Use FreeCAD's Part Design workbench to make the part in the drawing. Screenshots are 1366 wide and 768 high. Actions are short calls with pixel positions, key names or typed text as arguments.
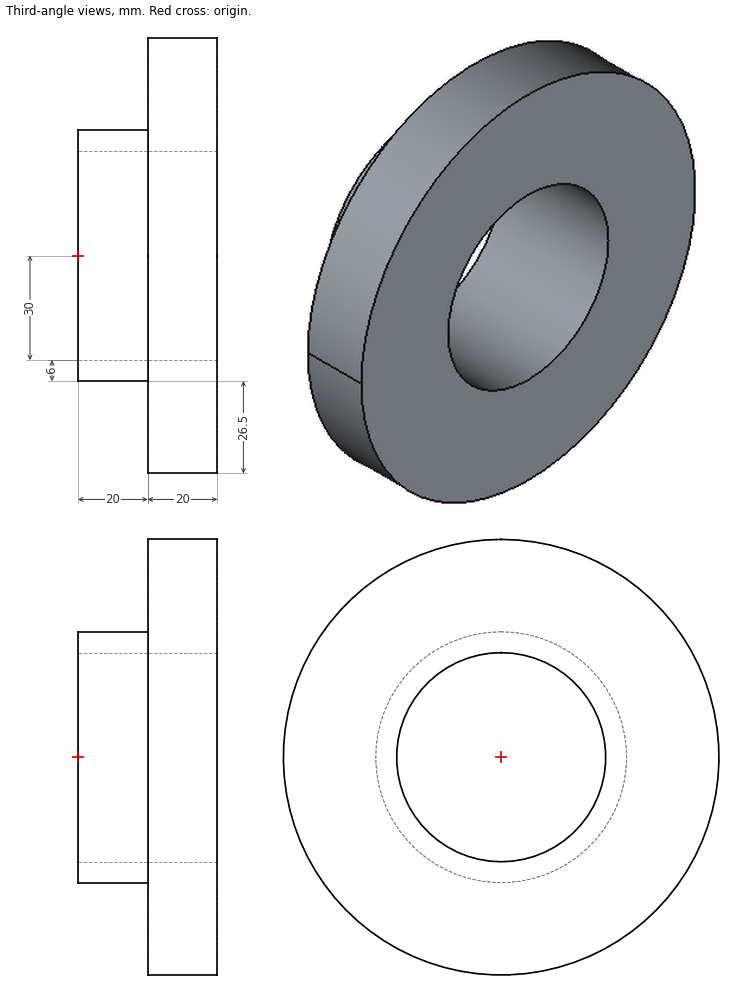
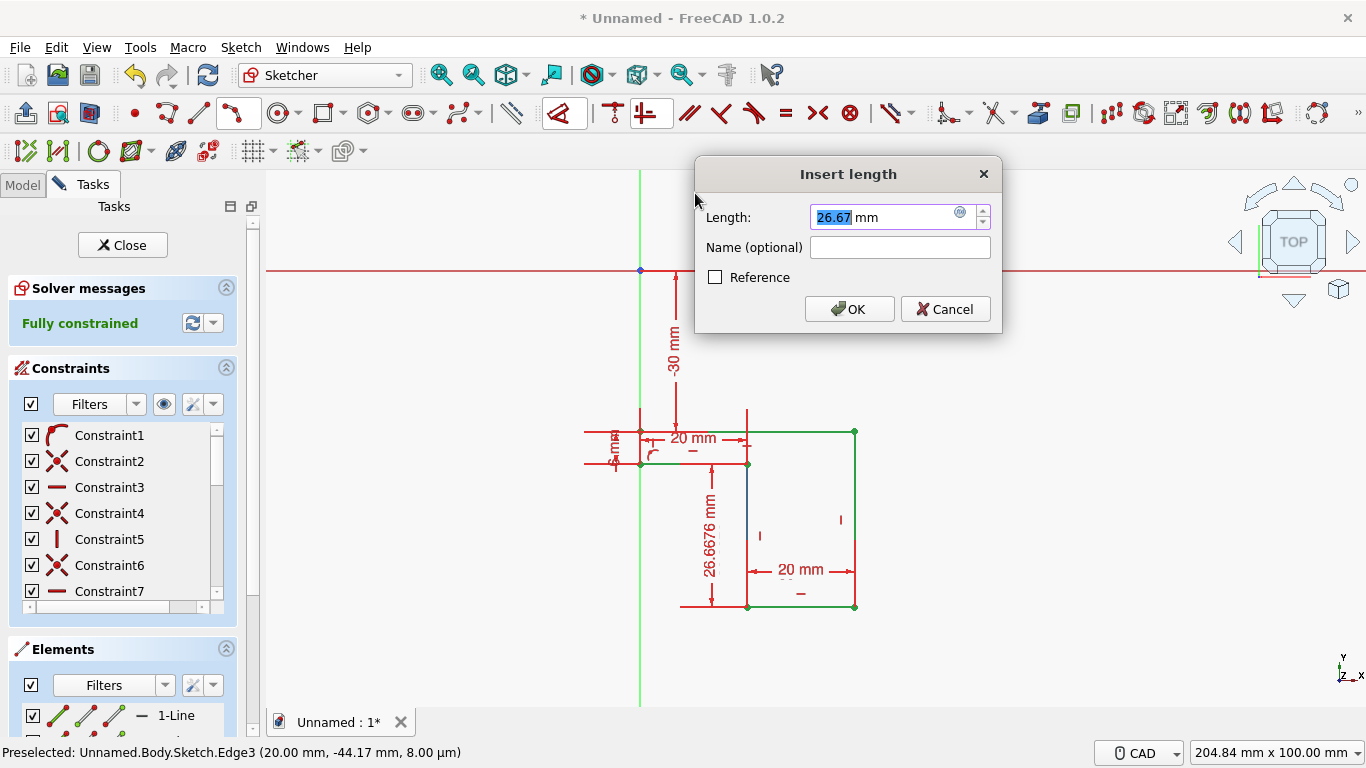
text(26.5)
key(Return)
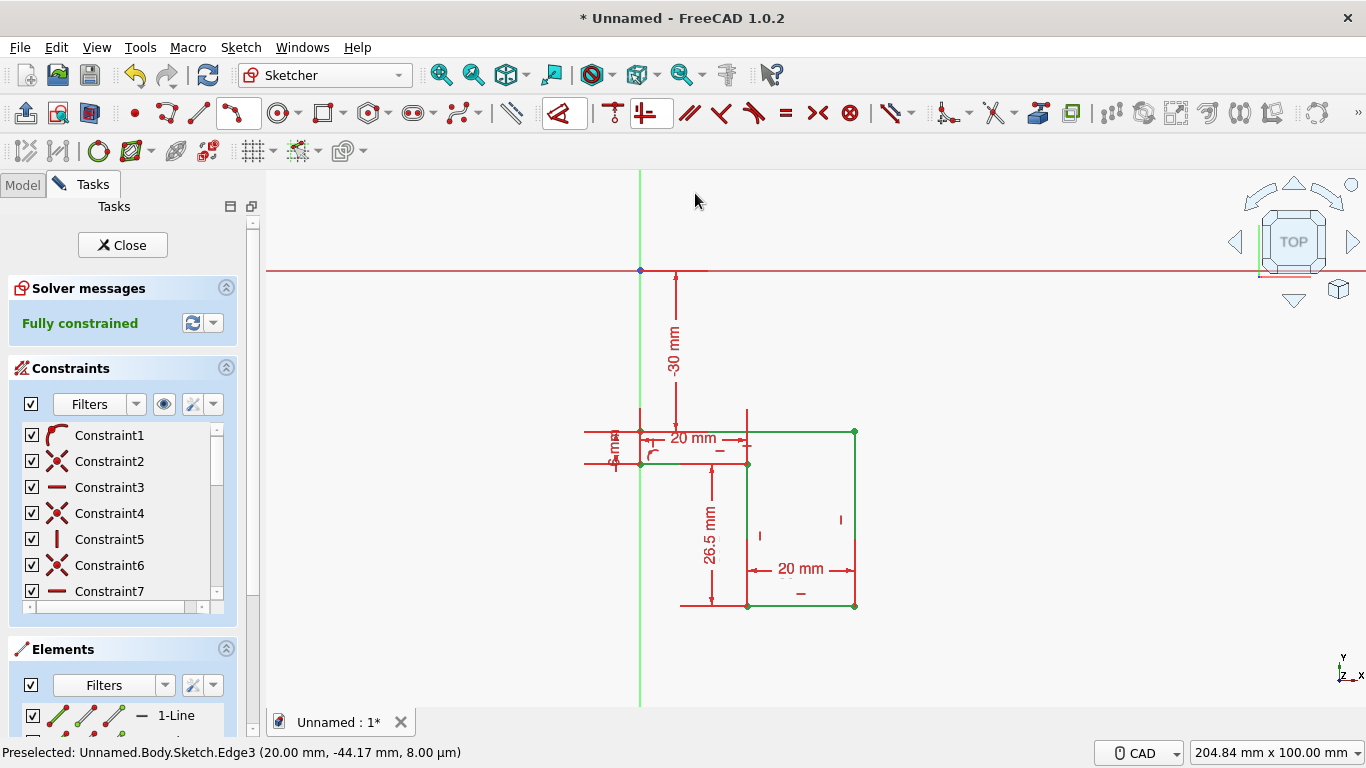
click(123, 245)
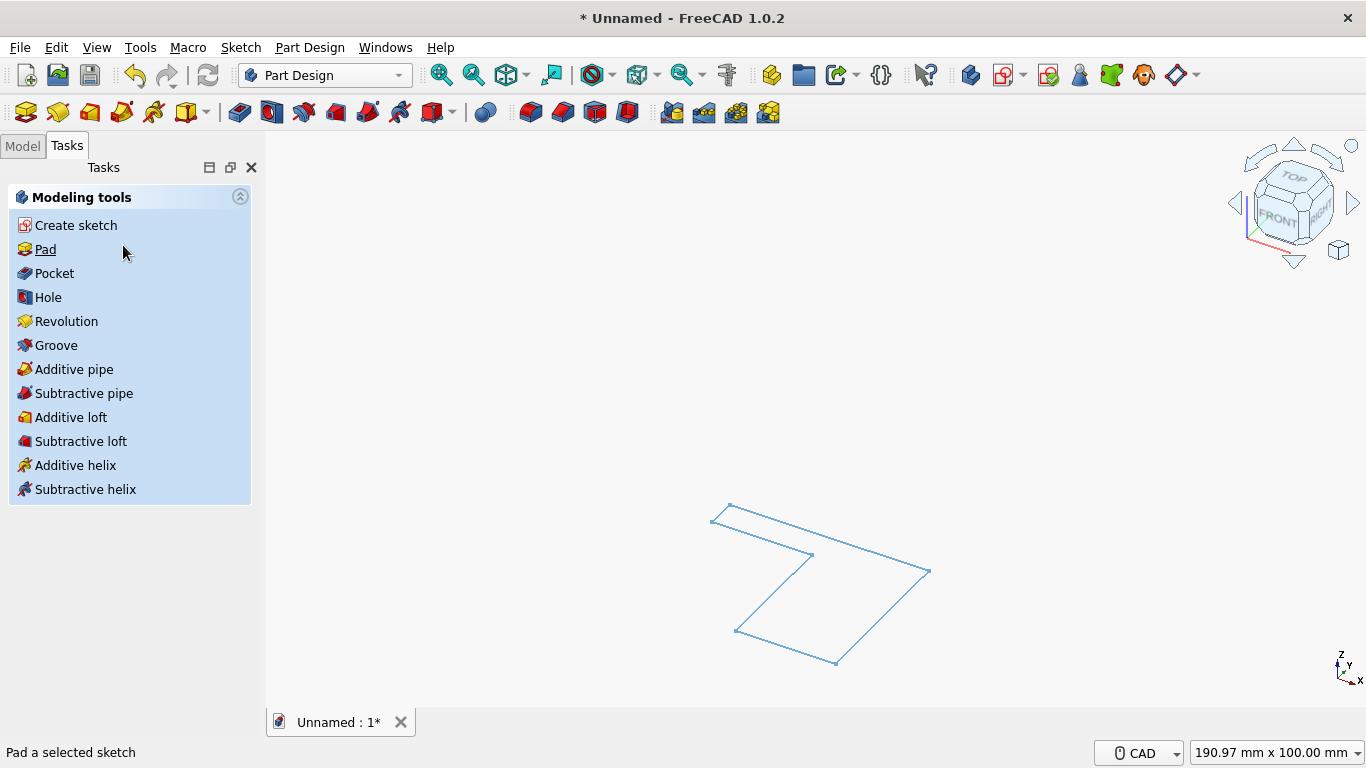
click(58, 112)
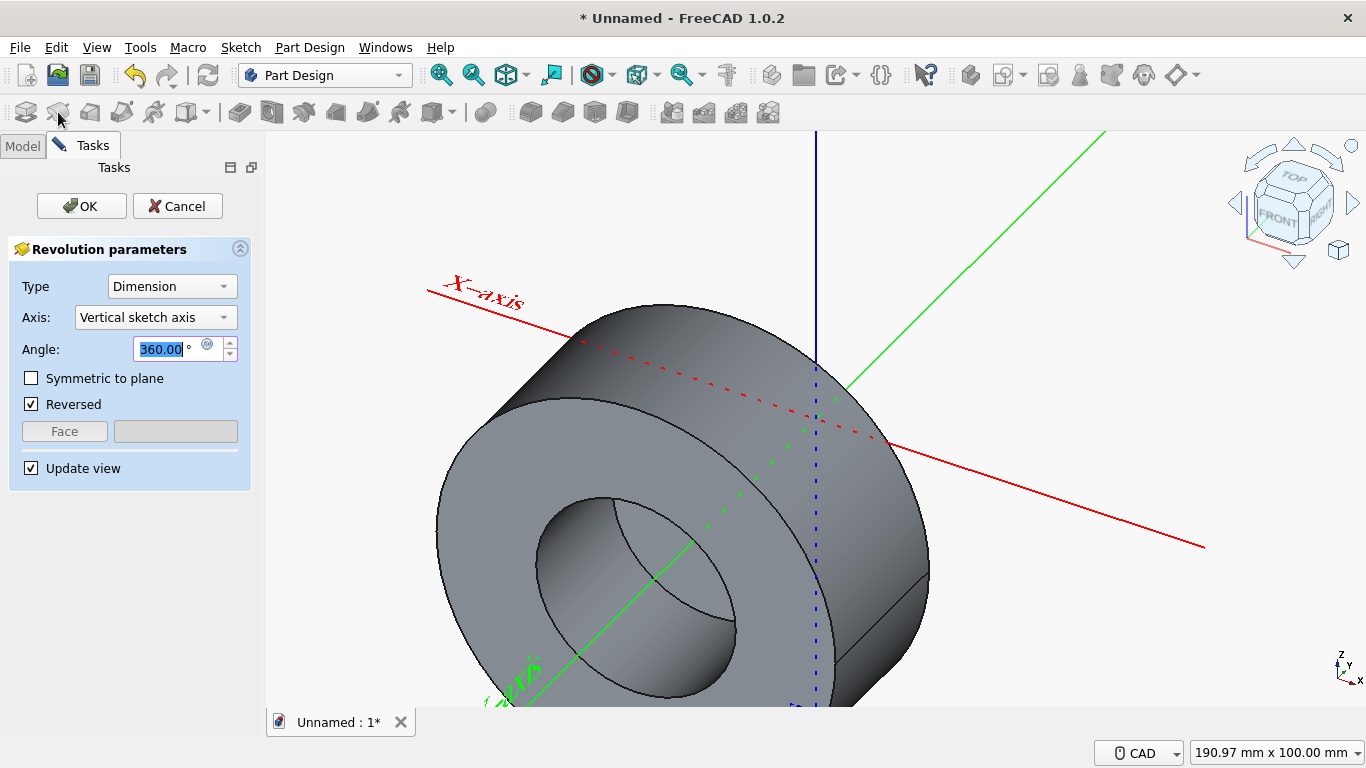
click(156, 318)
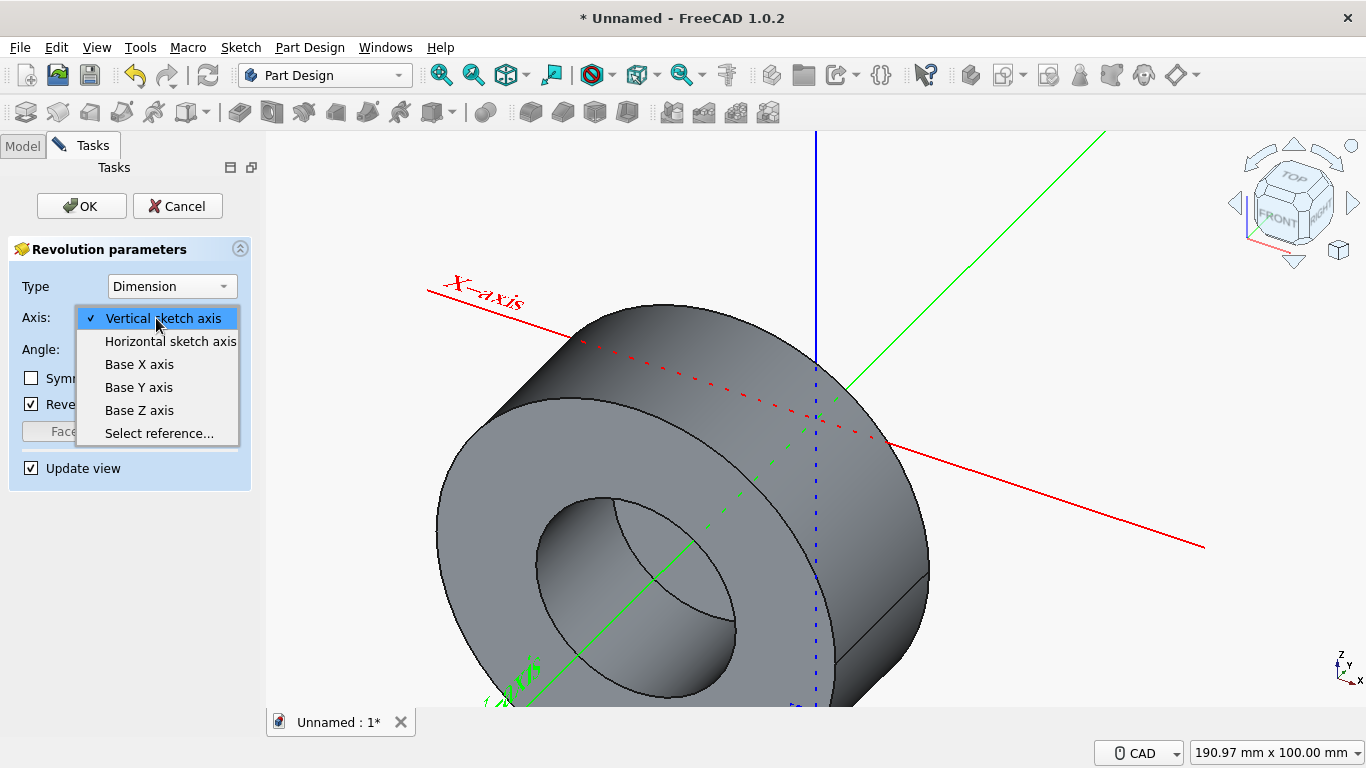
click(156, 342)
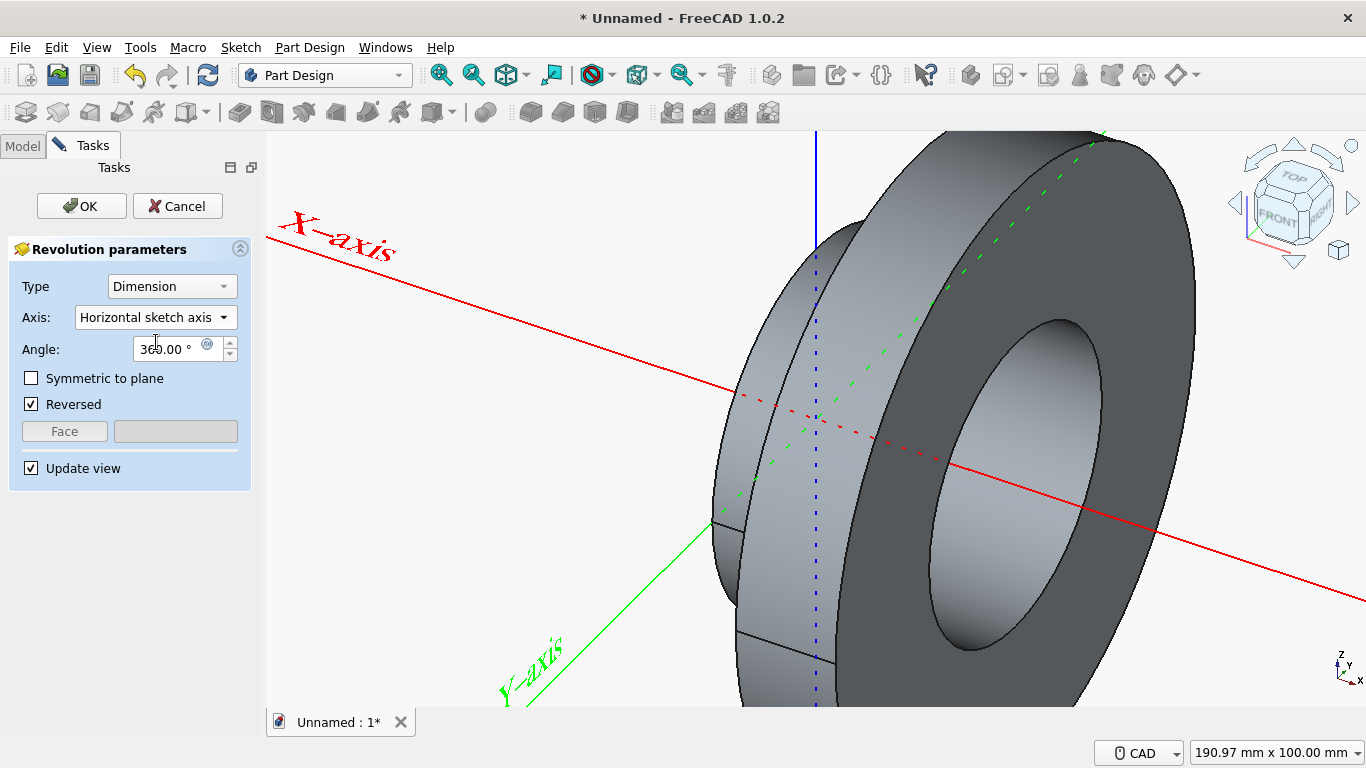
click(82, 206)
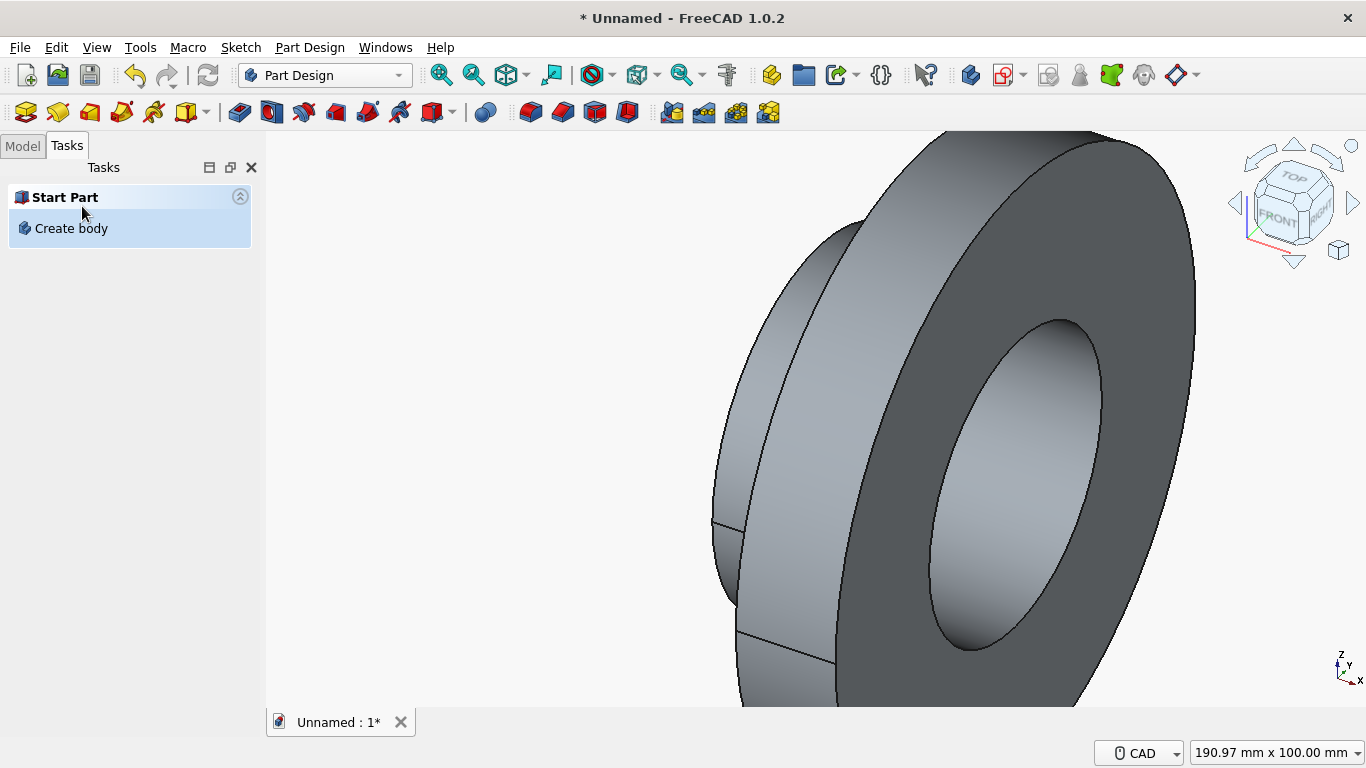
key(0)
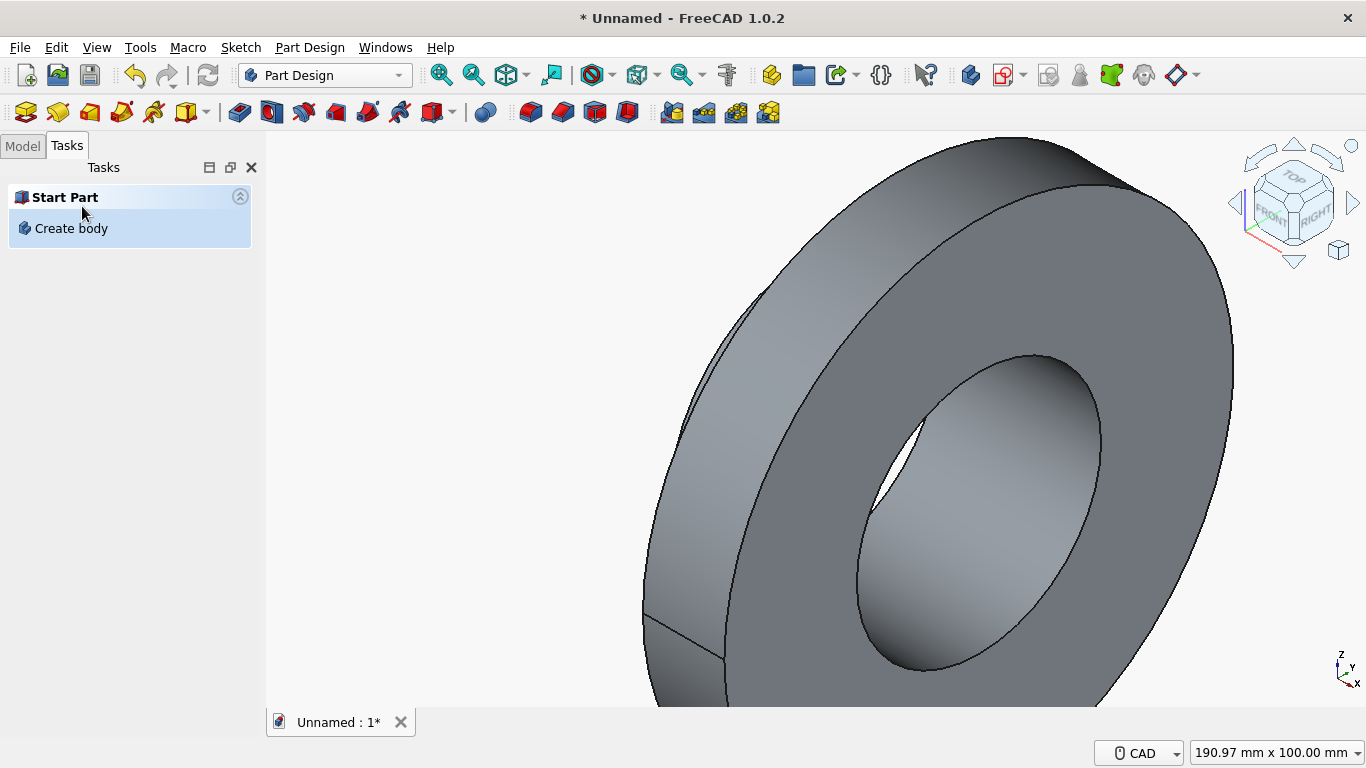
click(442, 76)